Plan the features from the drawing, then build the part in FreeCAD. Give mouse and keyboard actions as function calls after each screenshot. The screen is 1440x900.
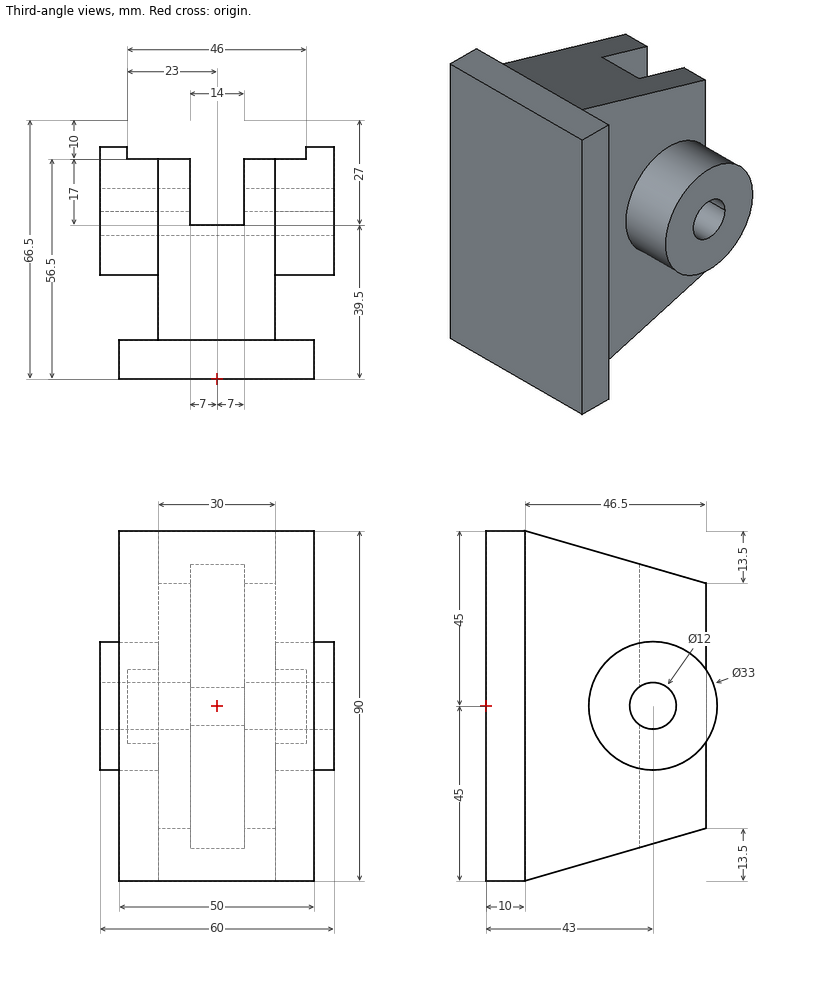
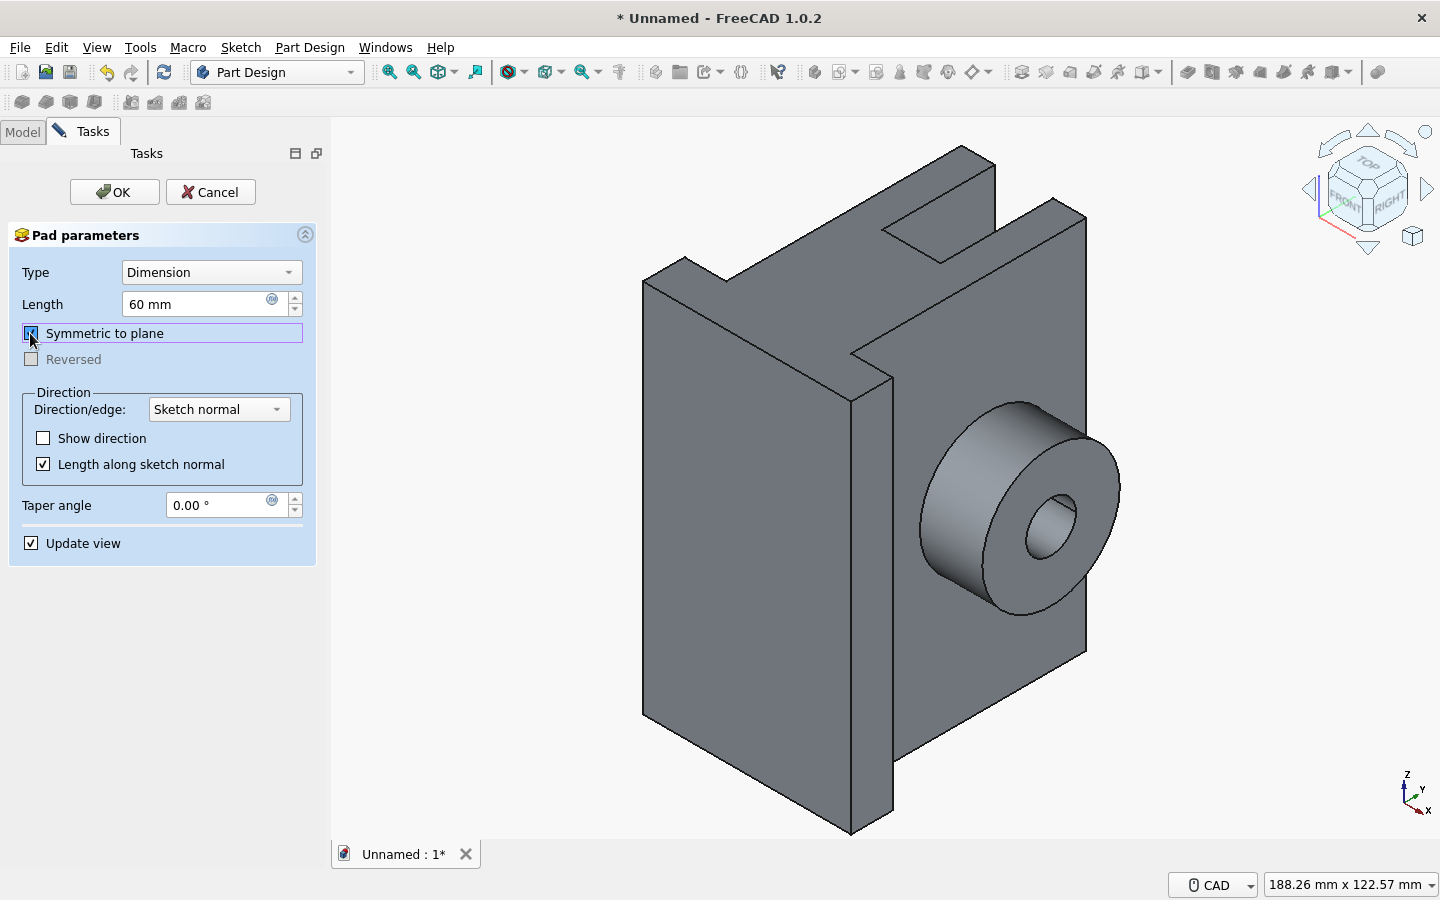
click(115, 192)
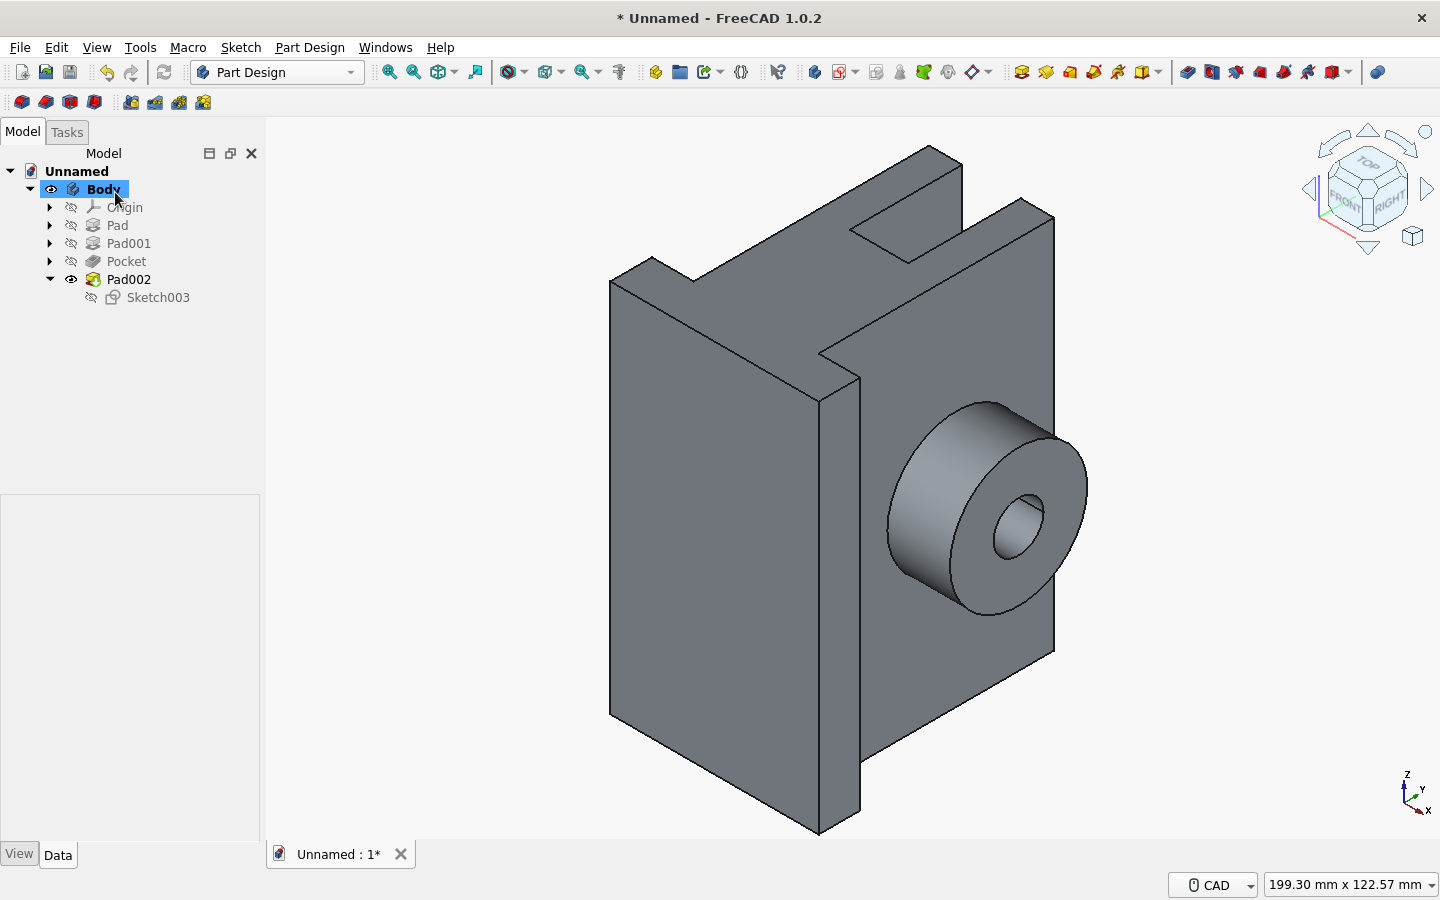
click(390, 72)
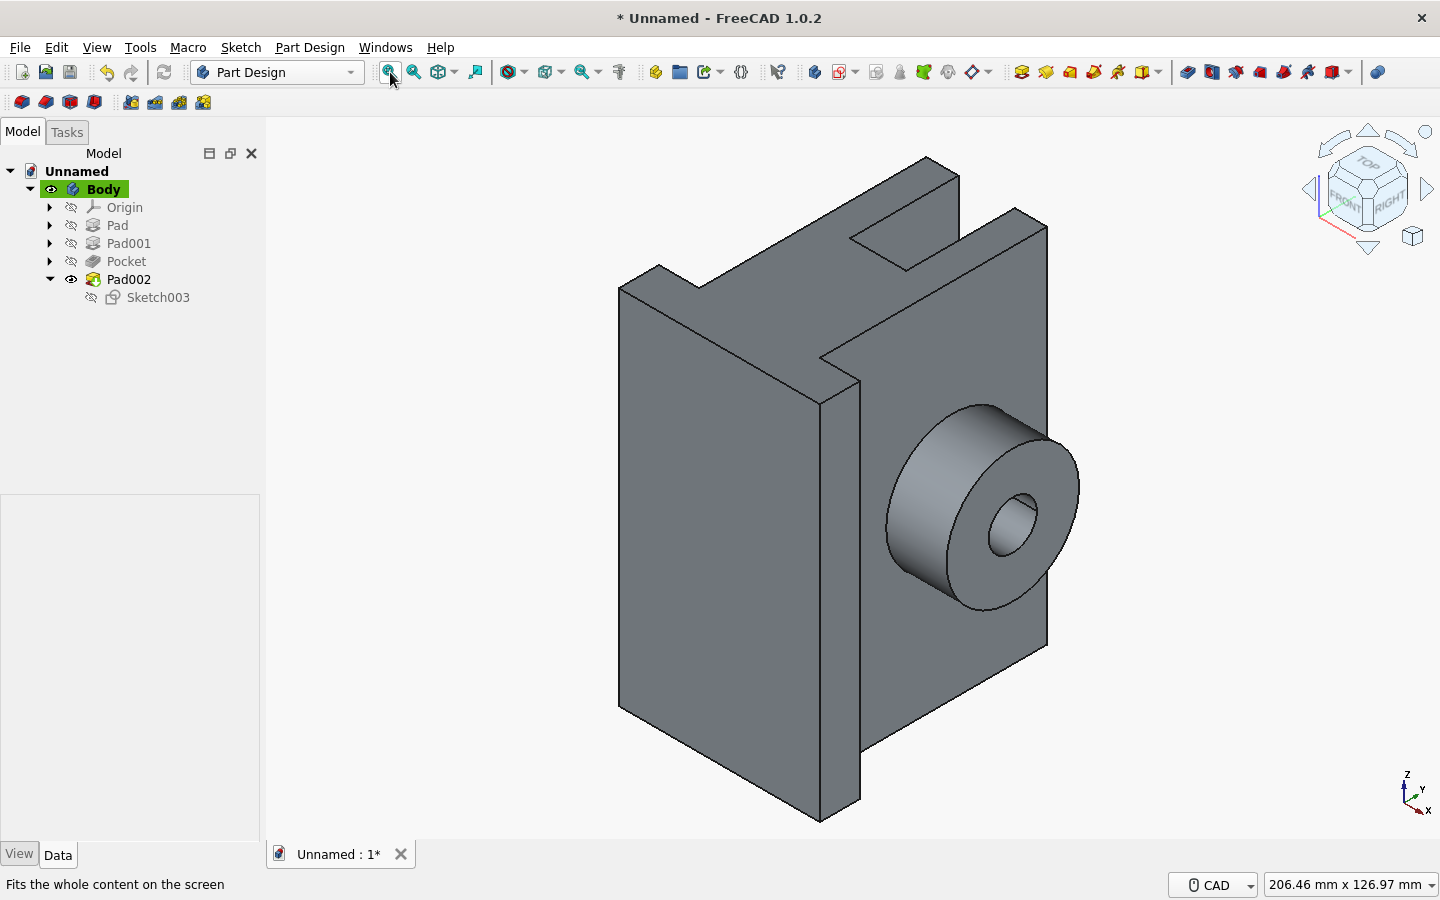
click(840, 72)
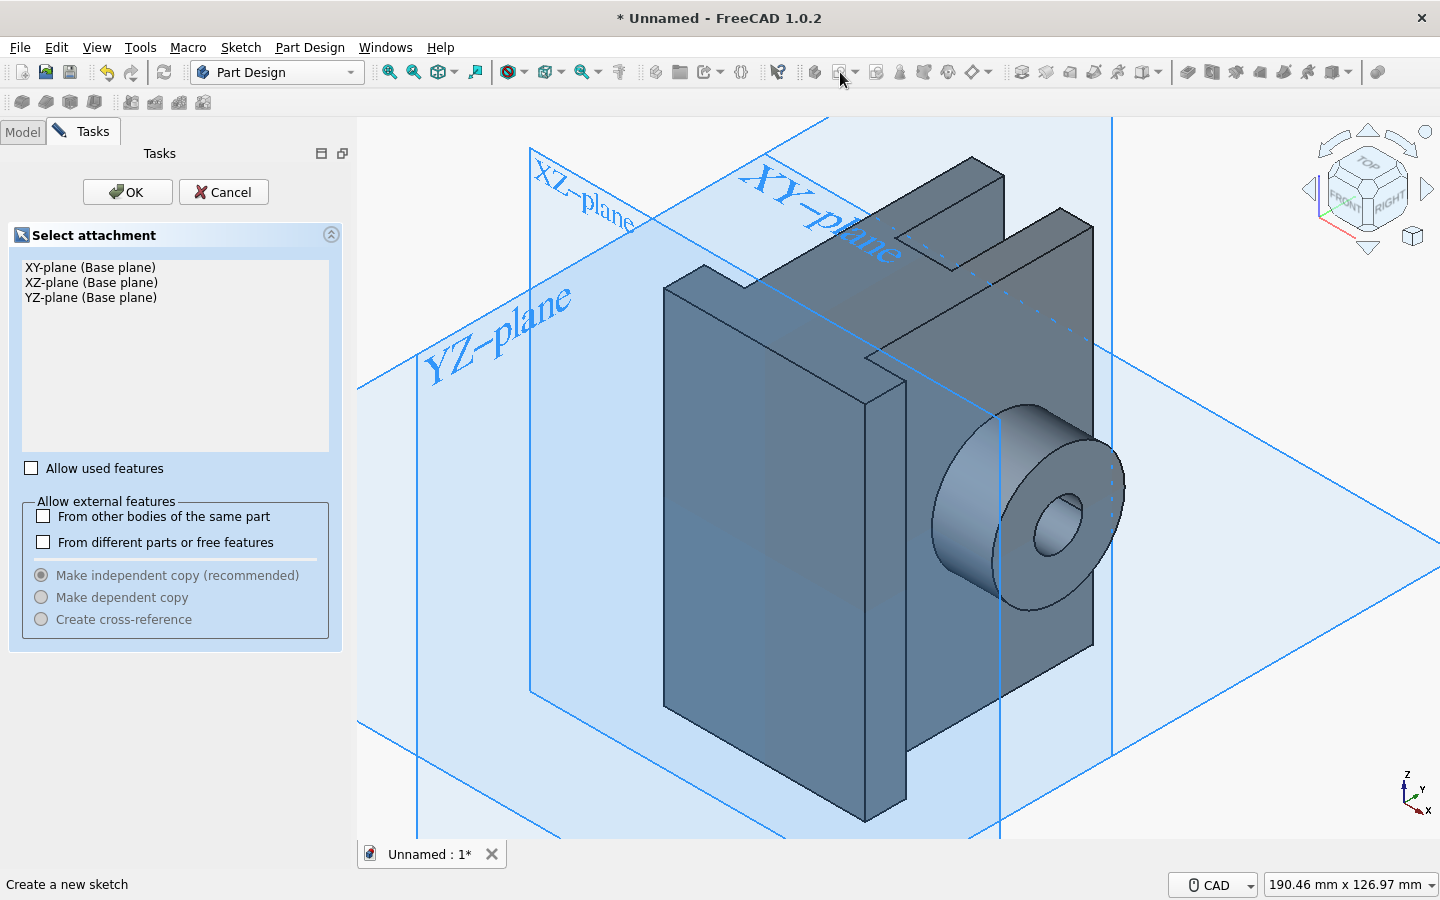
click(82, 268)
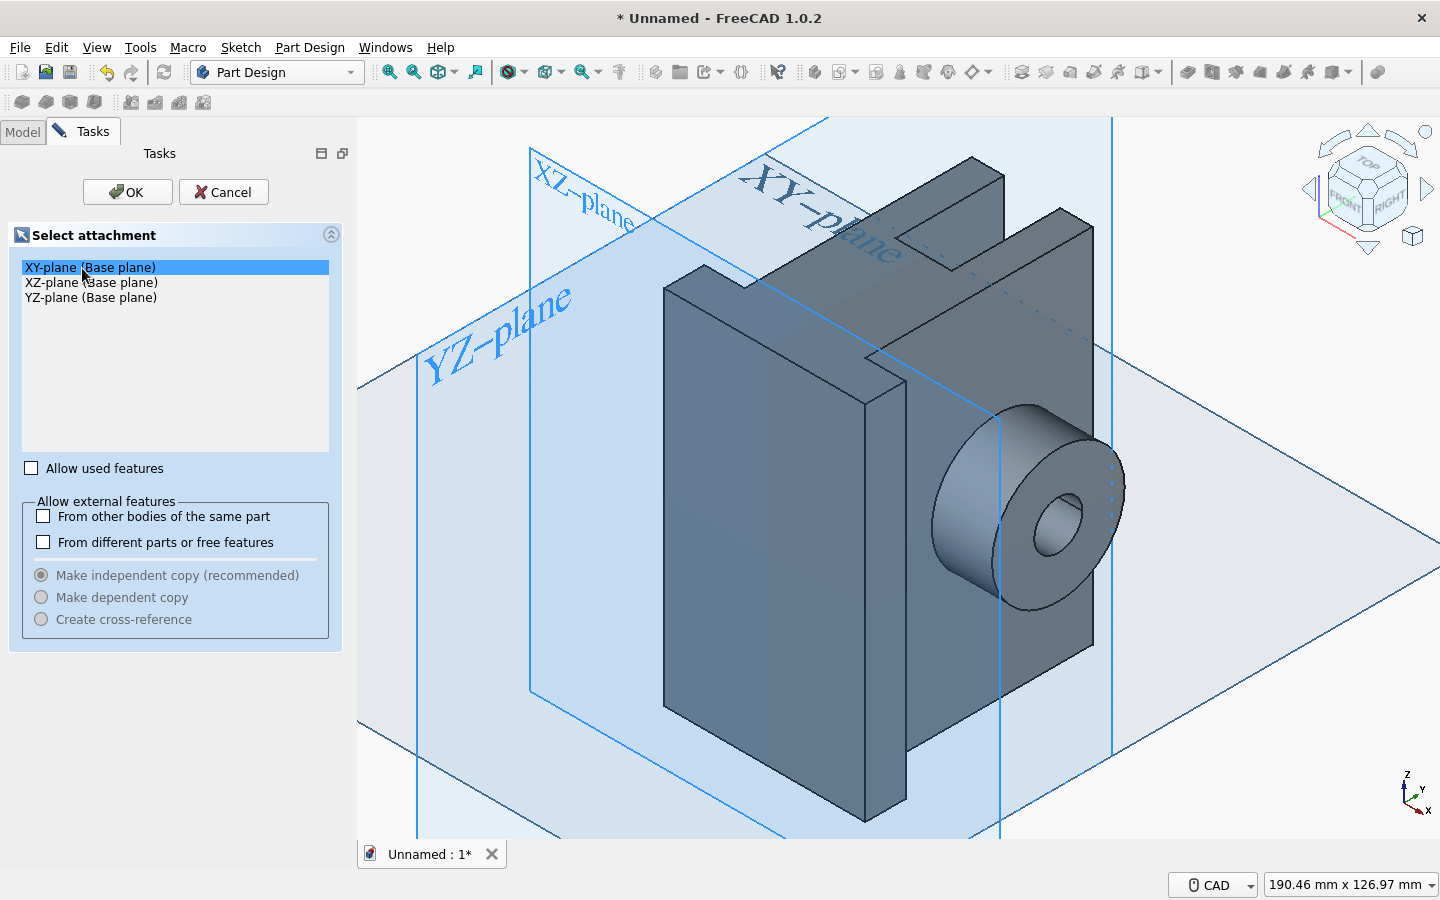
click(128, 192)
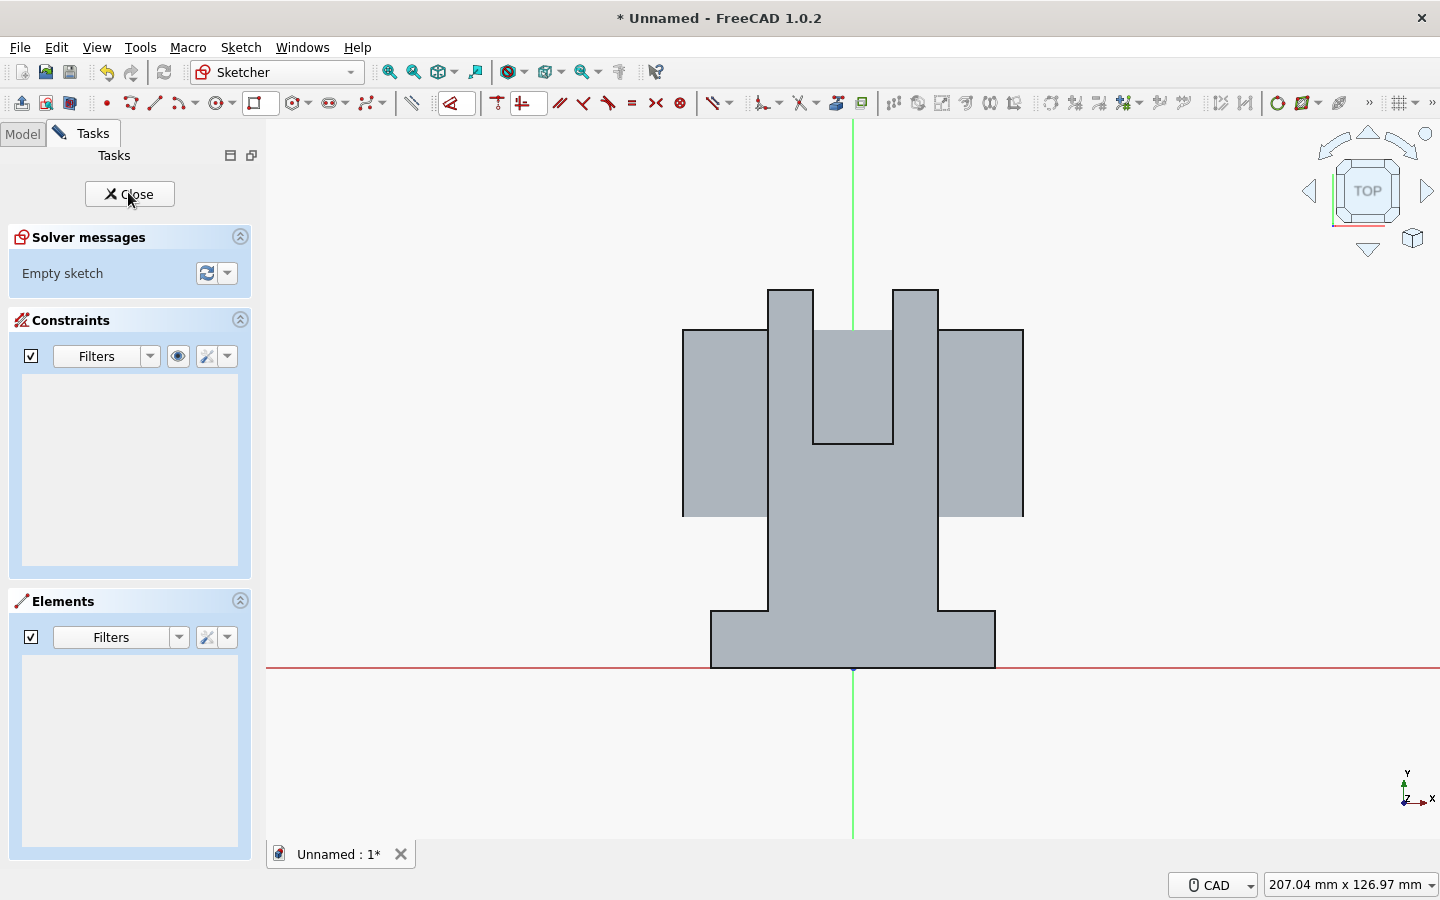
click(70, 104)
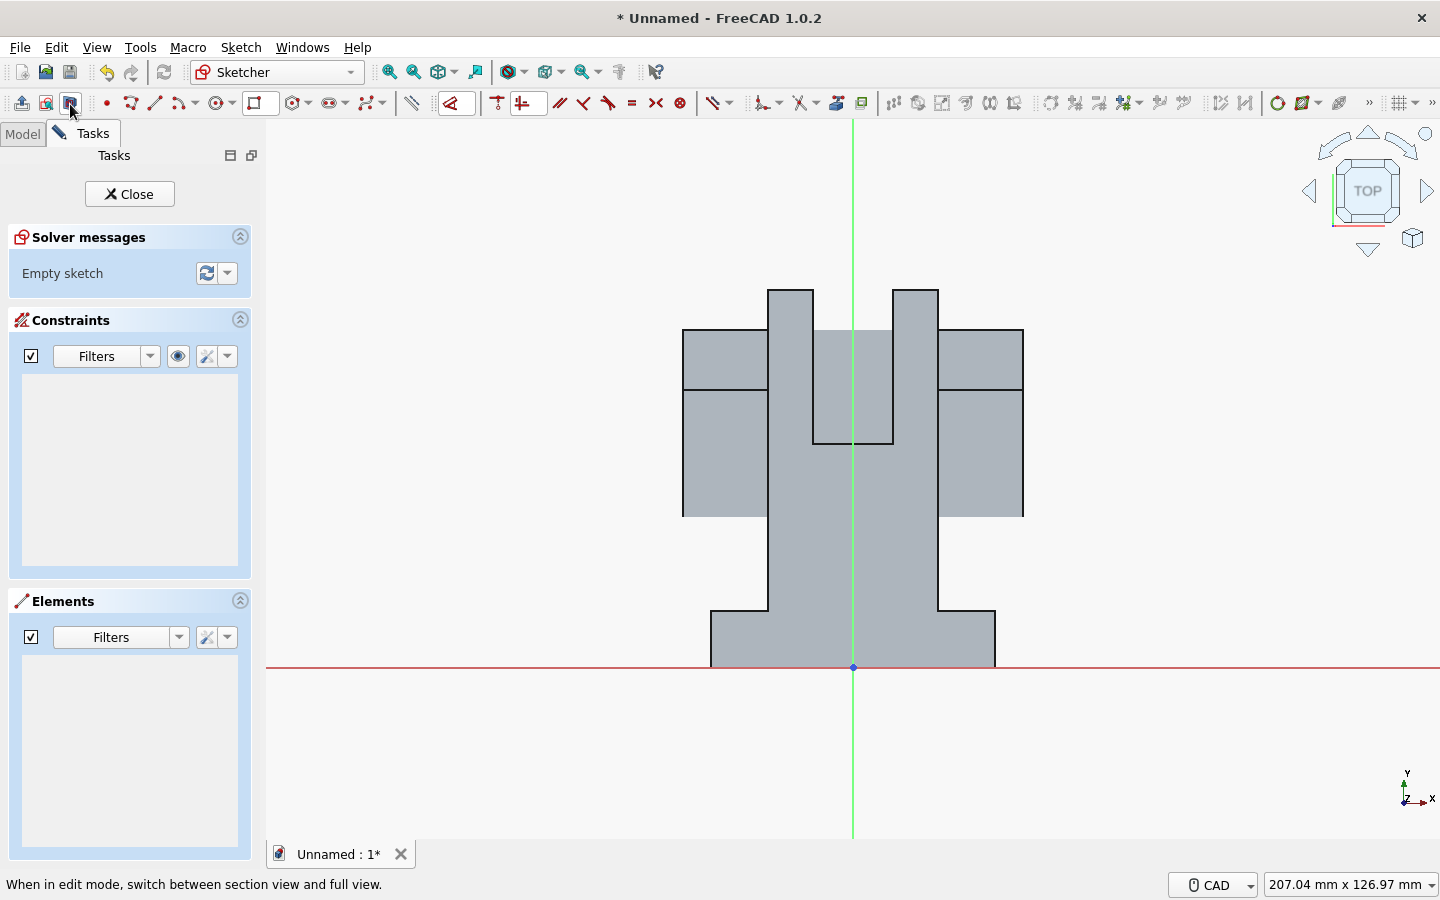
click(254, 104)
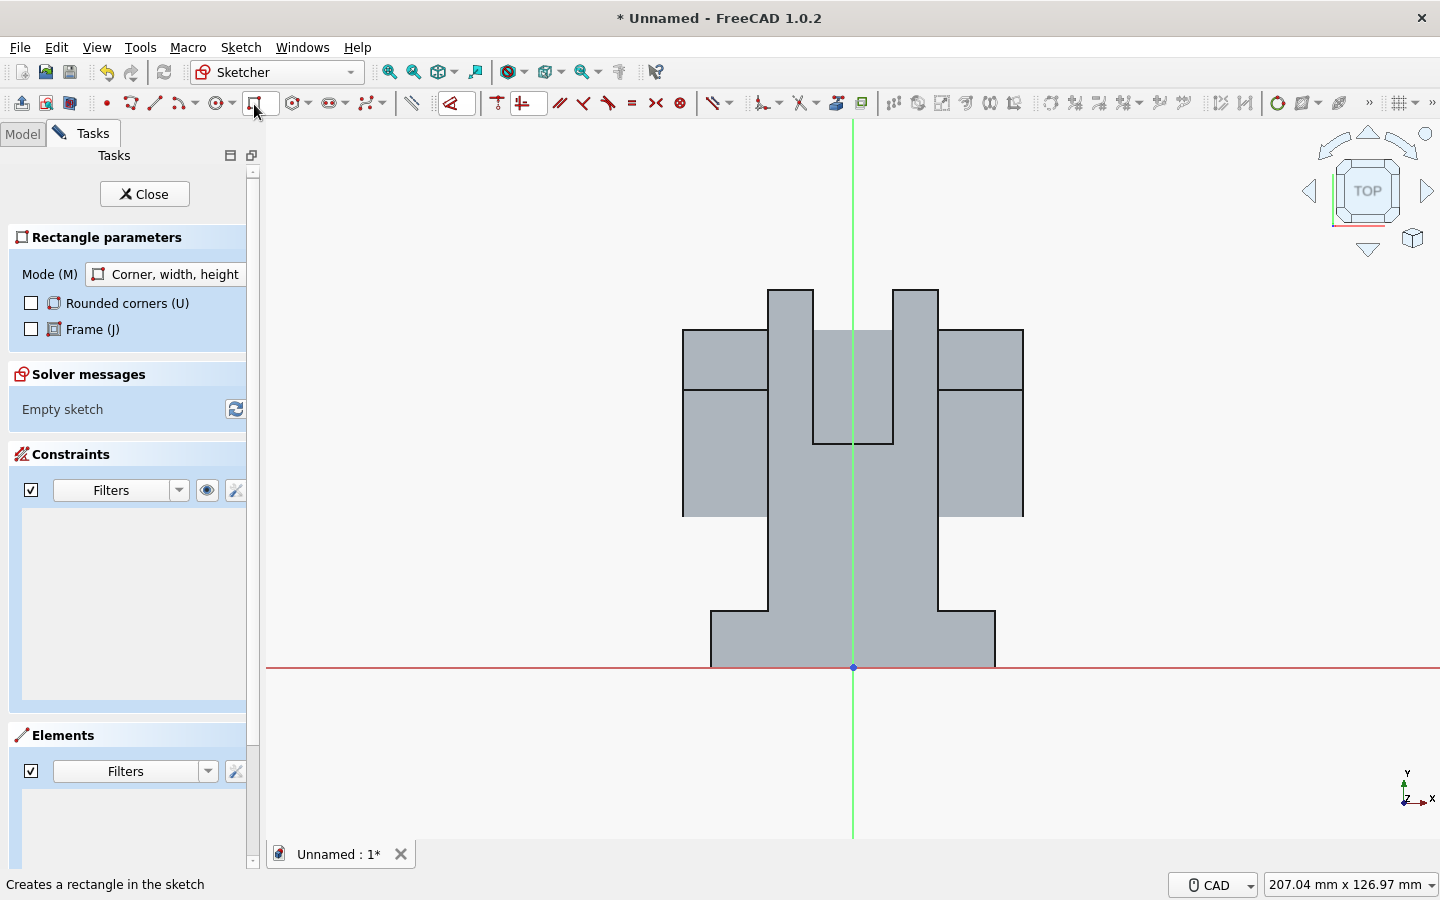
click(723, 290)
click(983, 347)
key(Escape)